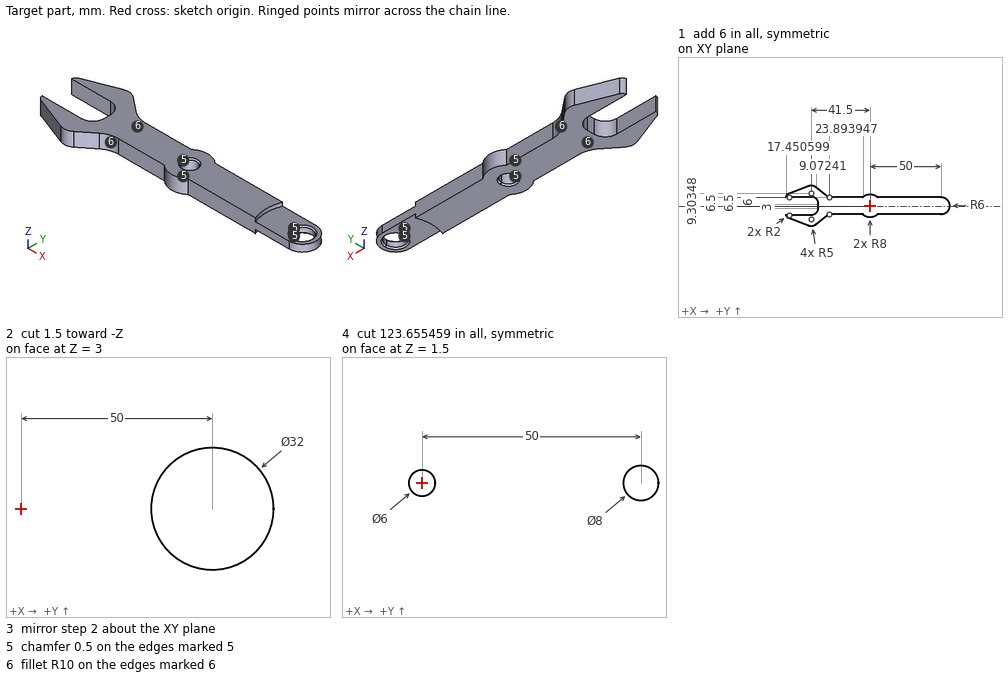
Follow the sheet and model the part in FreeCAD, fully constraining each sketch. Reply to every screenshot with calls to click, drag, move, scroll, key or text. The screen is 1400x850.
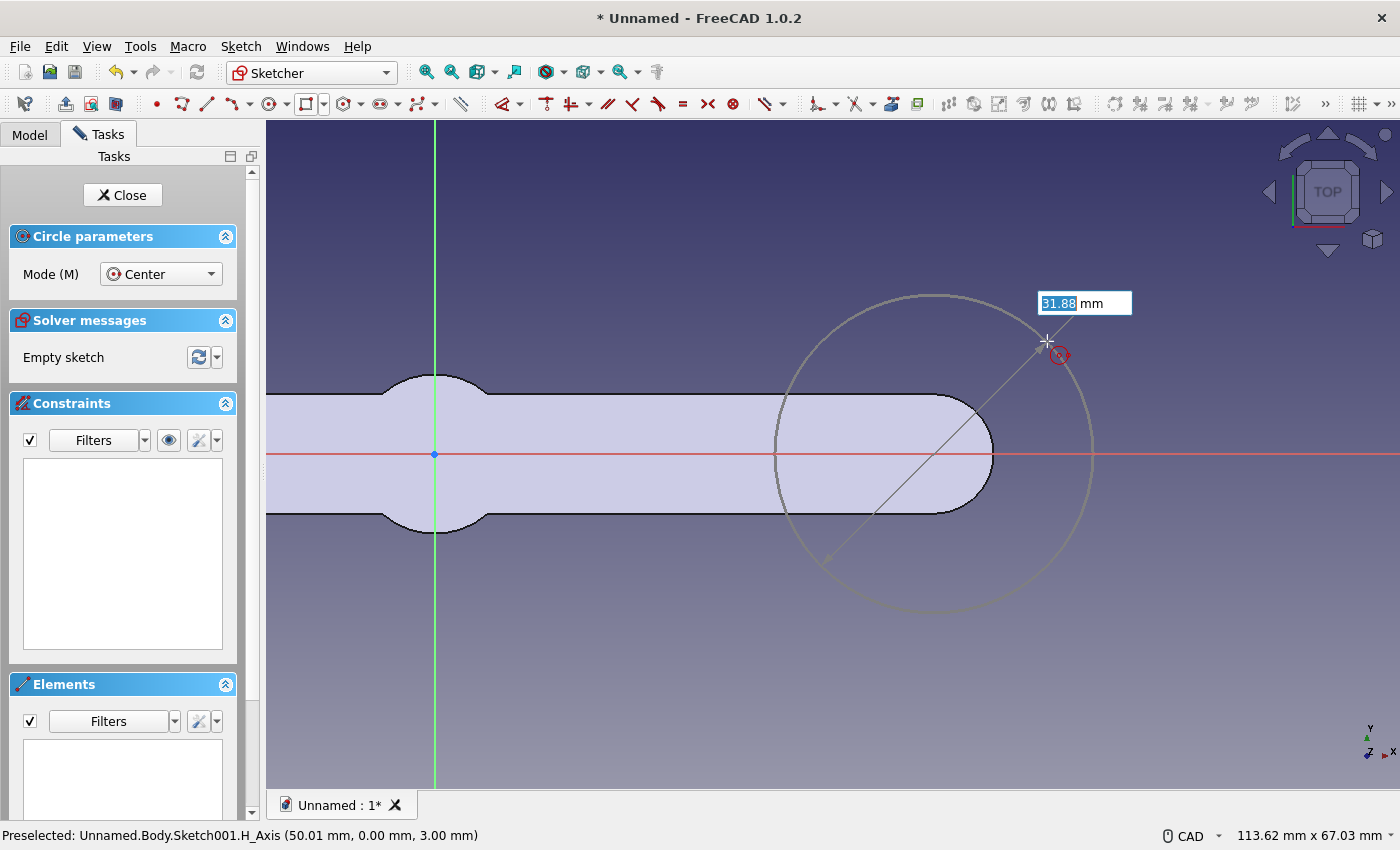
text(32)
key(Return)
key(Escape)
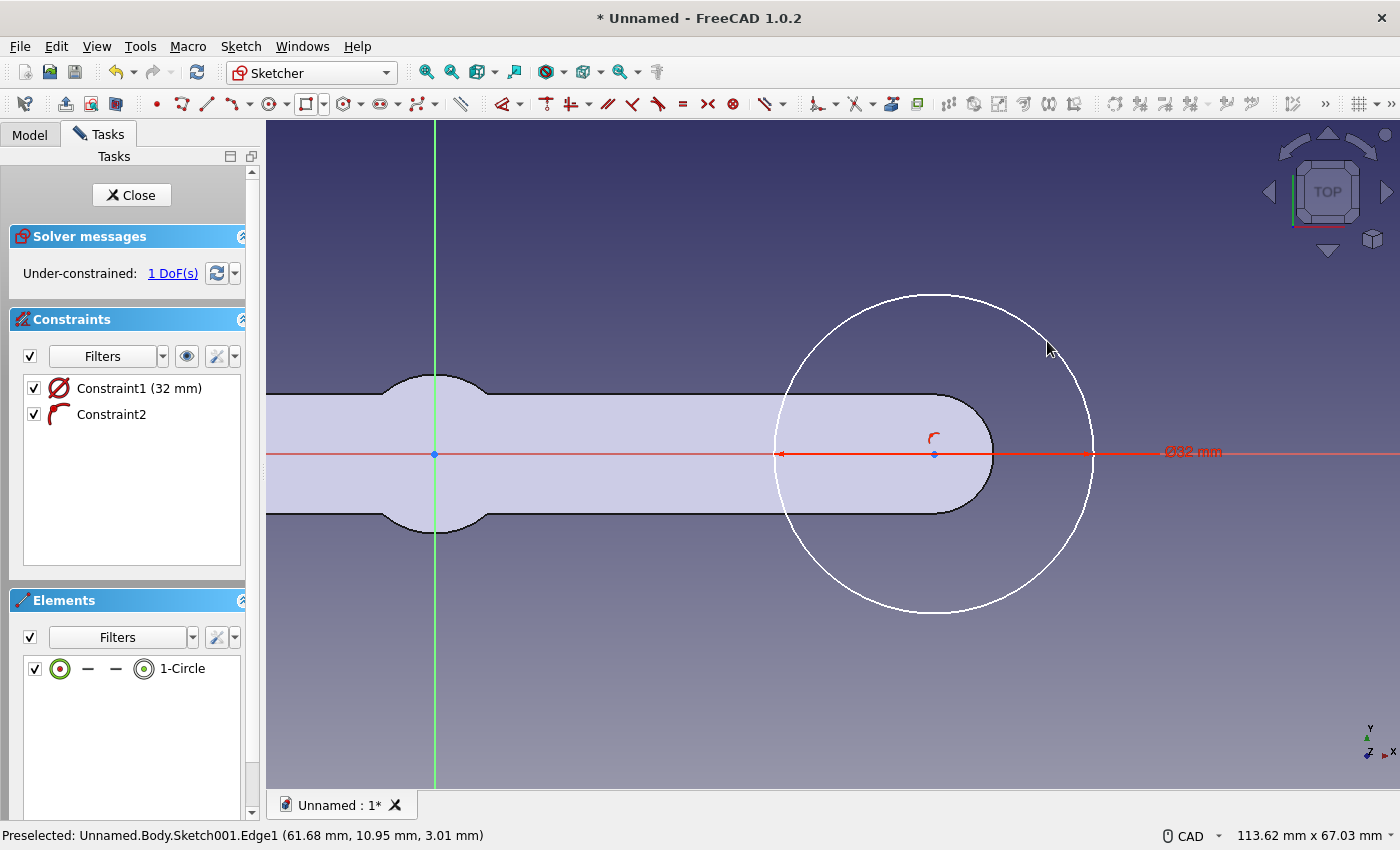
click(502, 104)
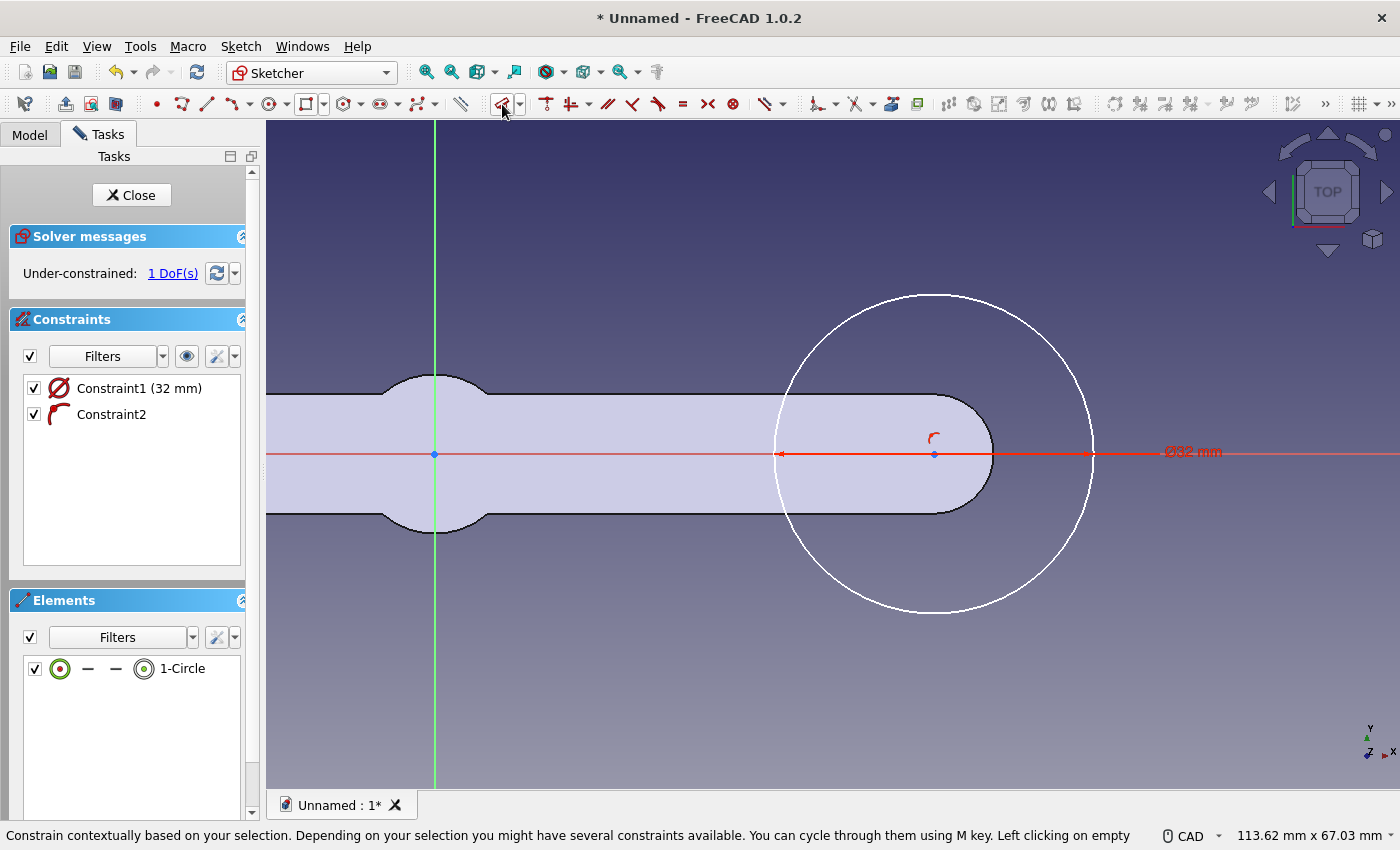
click(934, 454)
click(684, 488)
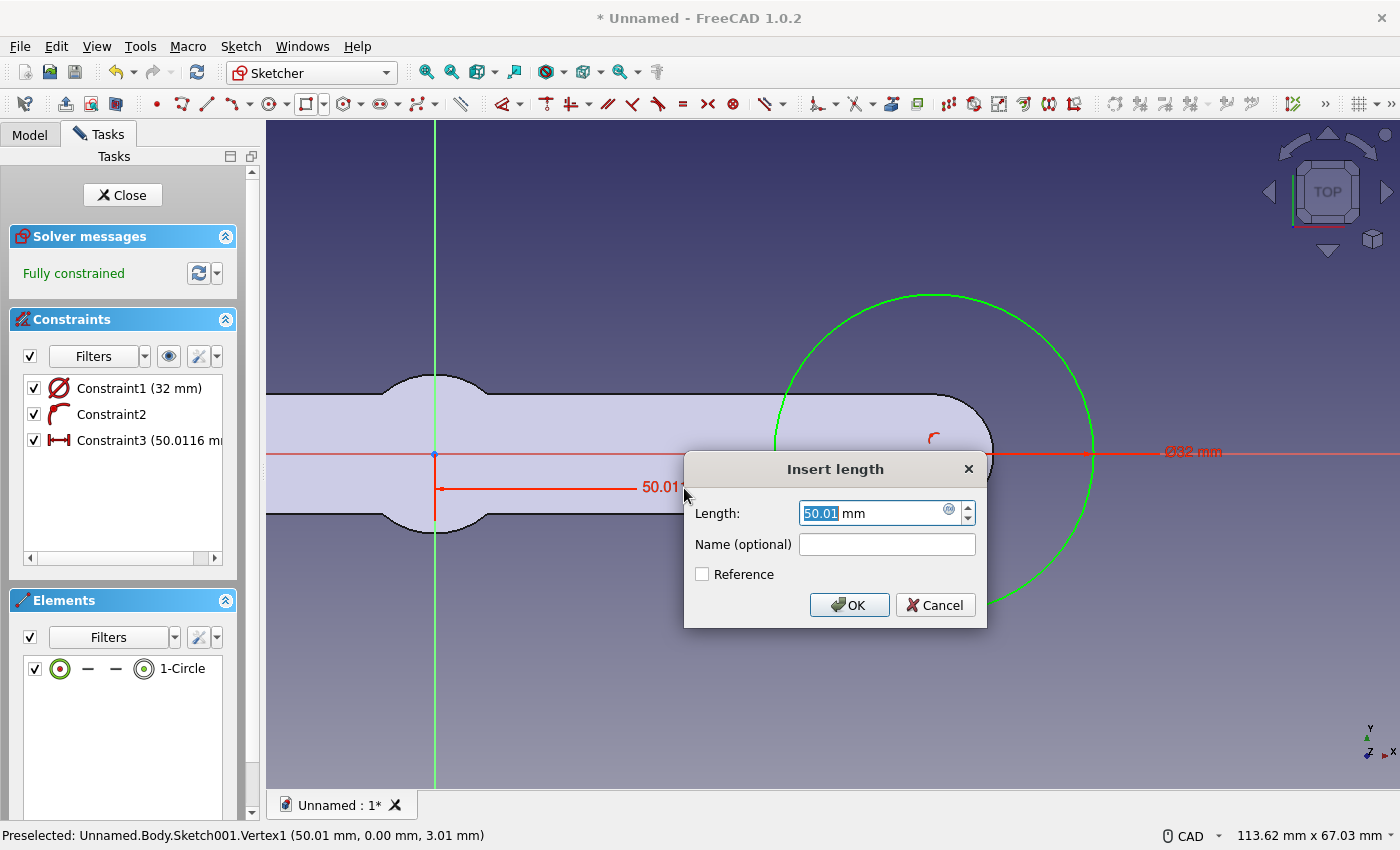
text(50)
key(Return)
key(Escape)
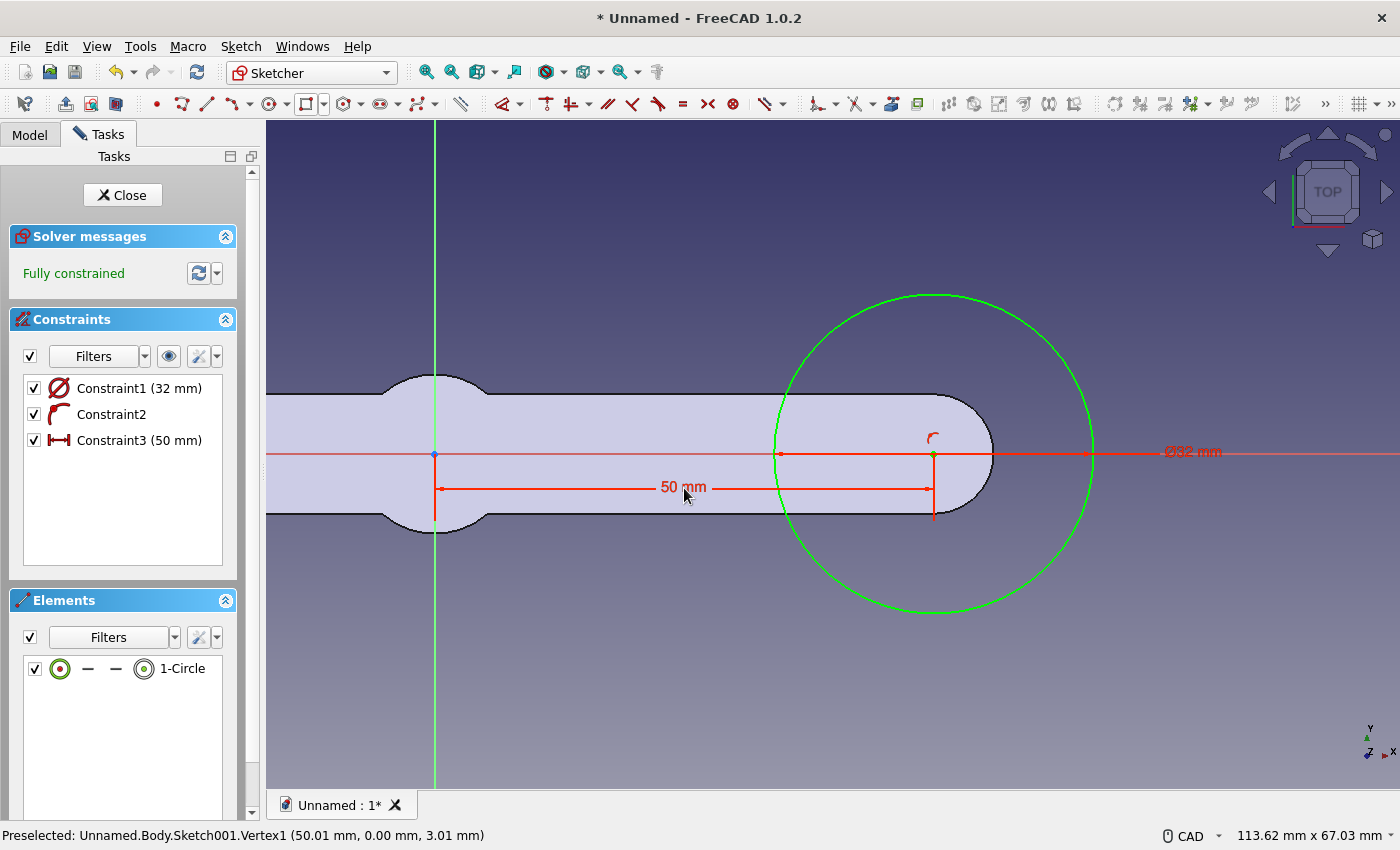
click(123, 195)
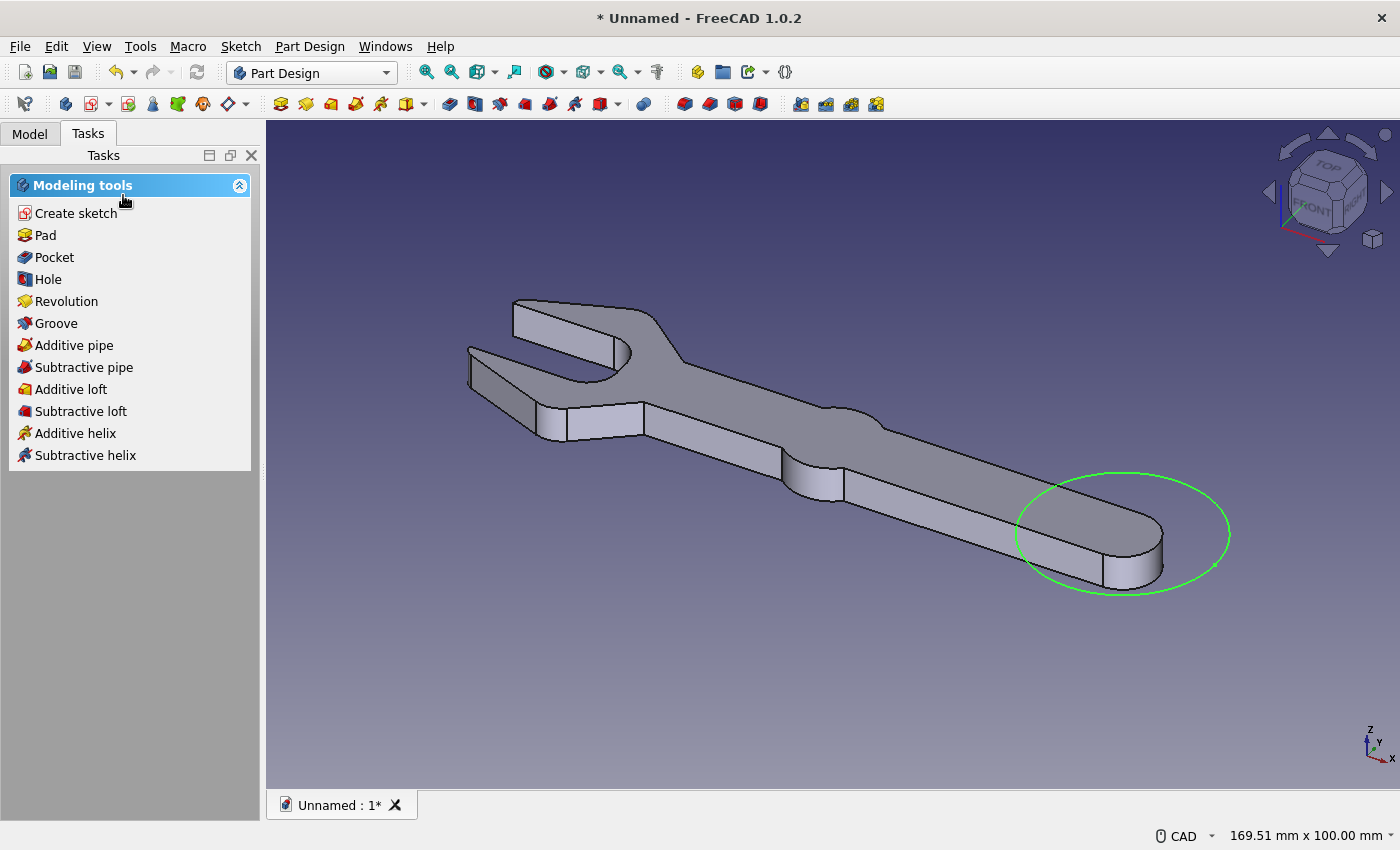
click(450, 104)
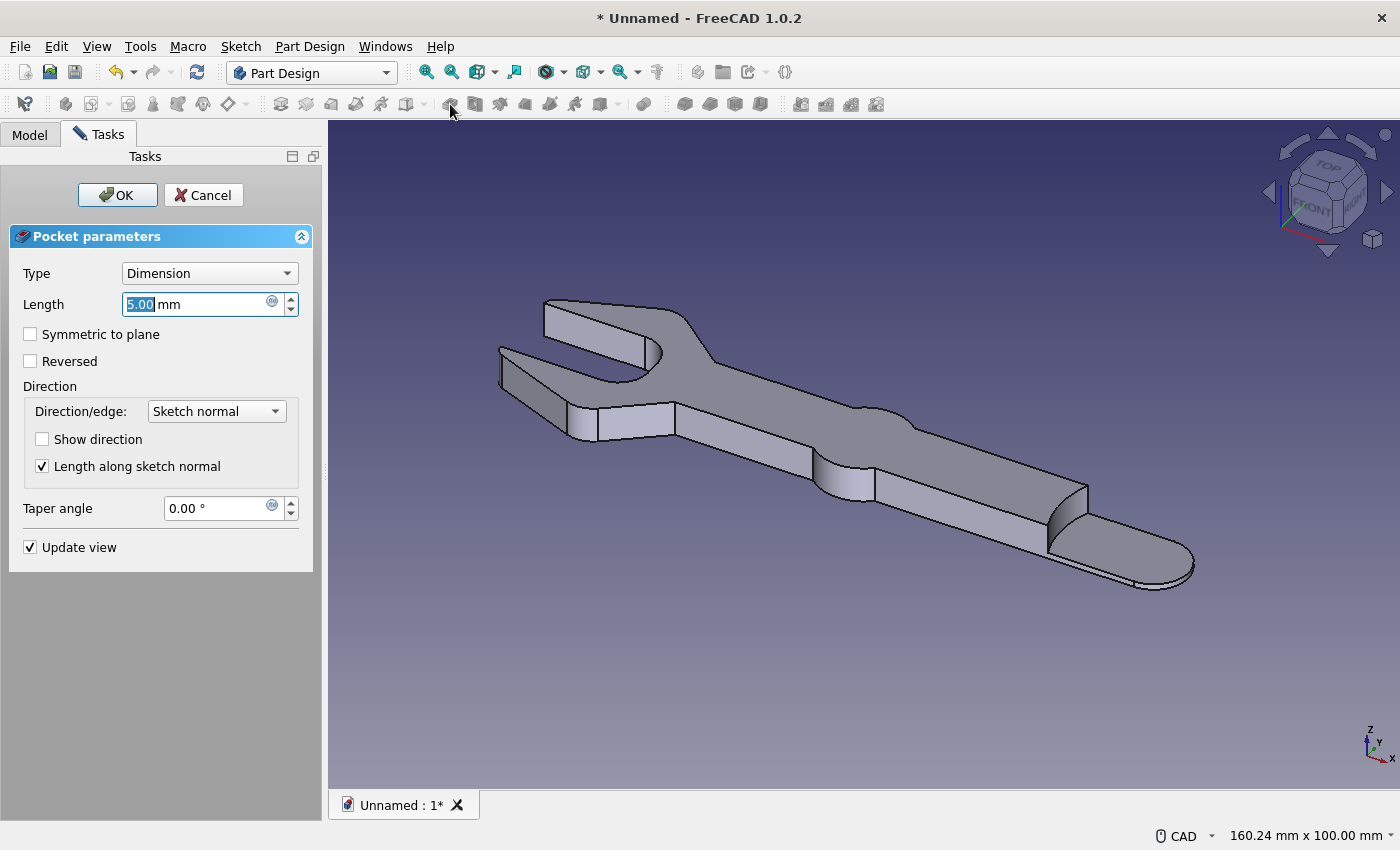
text(1.5)
key(Tab)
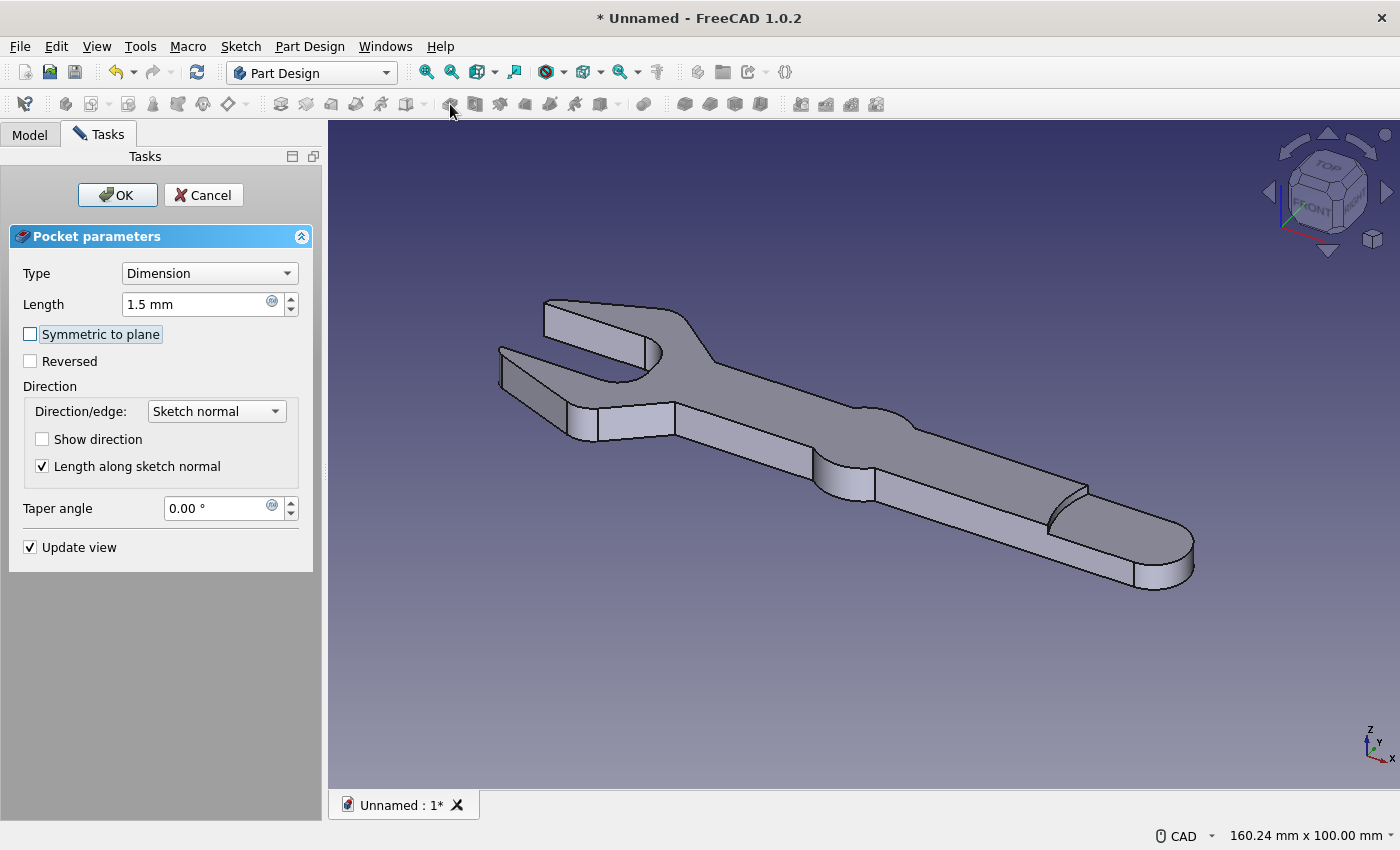
click(118, 195)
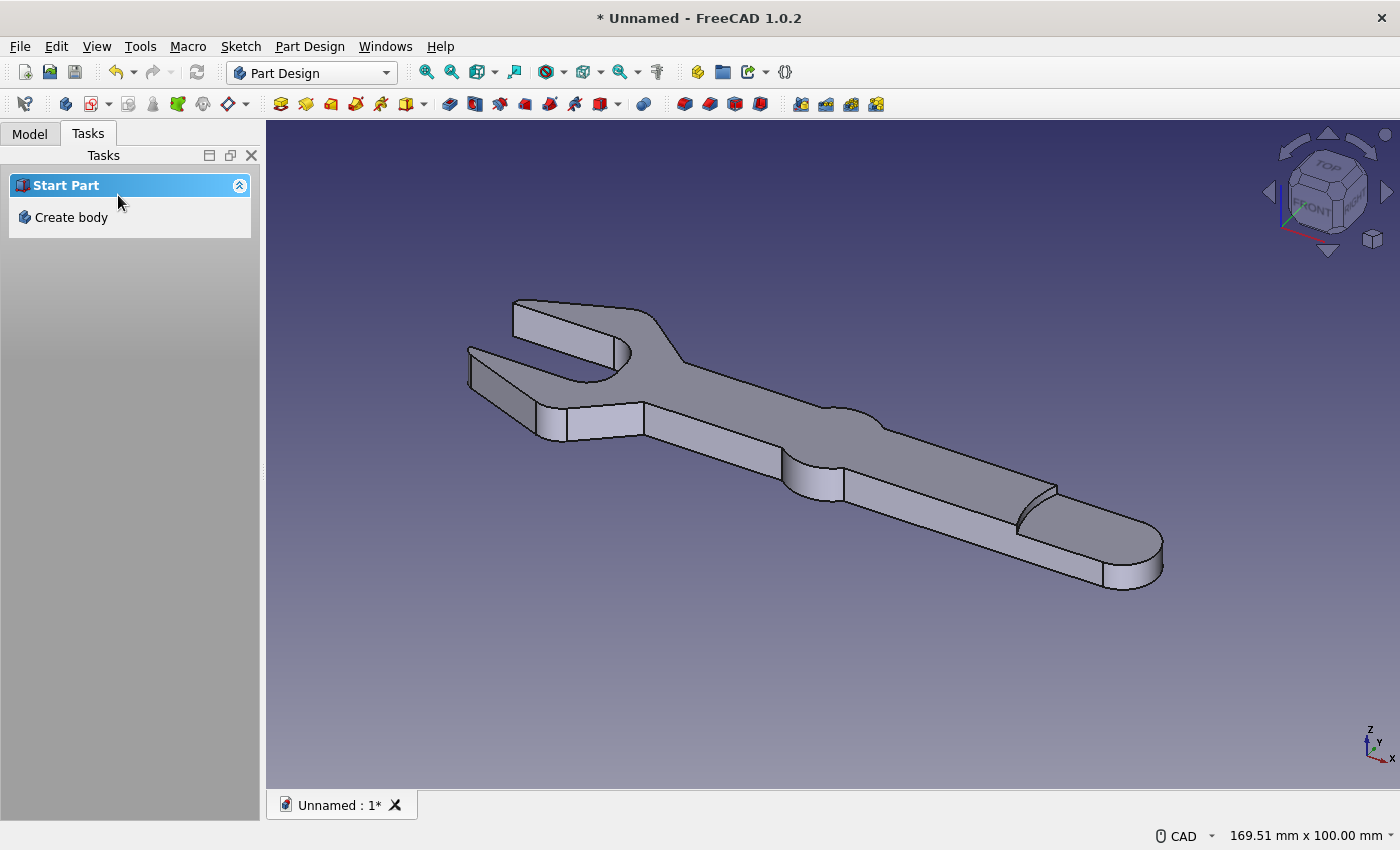
click(30, 134)